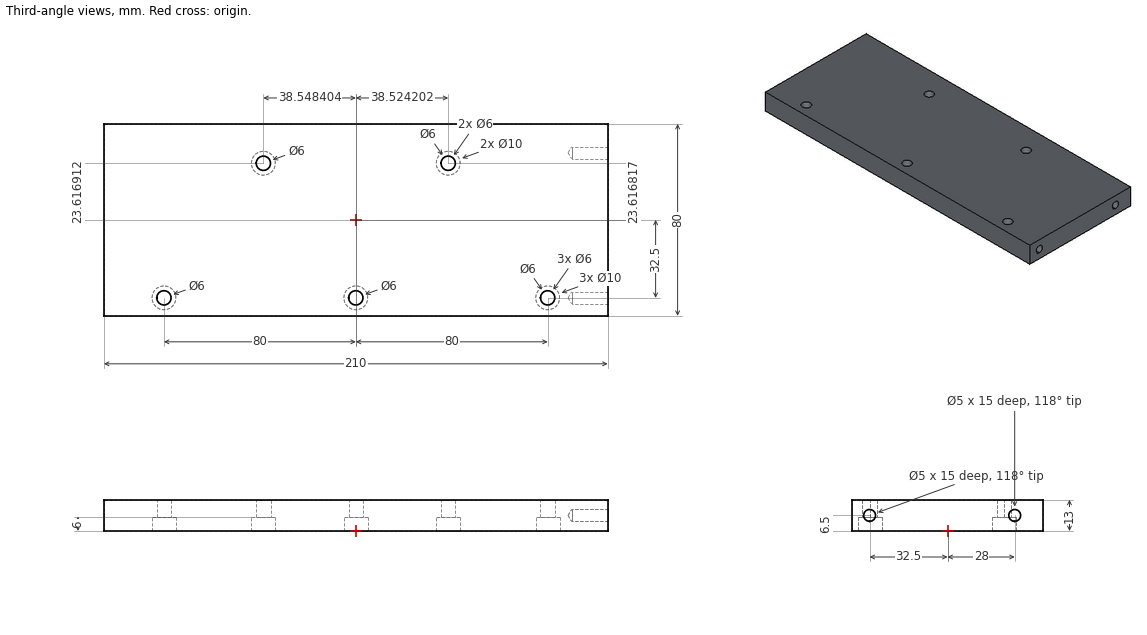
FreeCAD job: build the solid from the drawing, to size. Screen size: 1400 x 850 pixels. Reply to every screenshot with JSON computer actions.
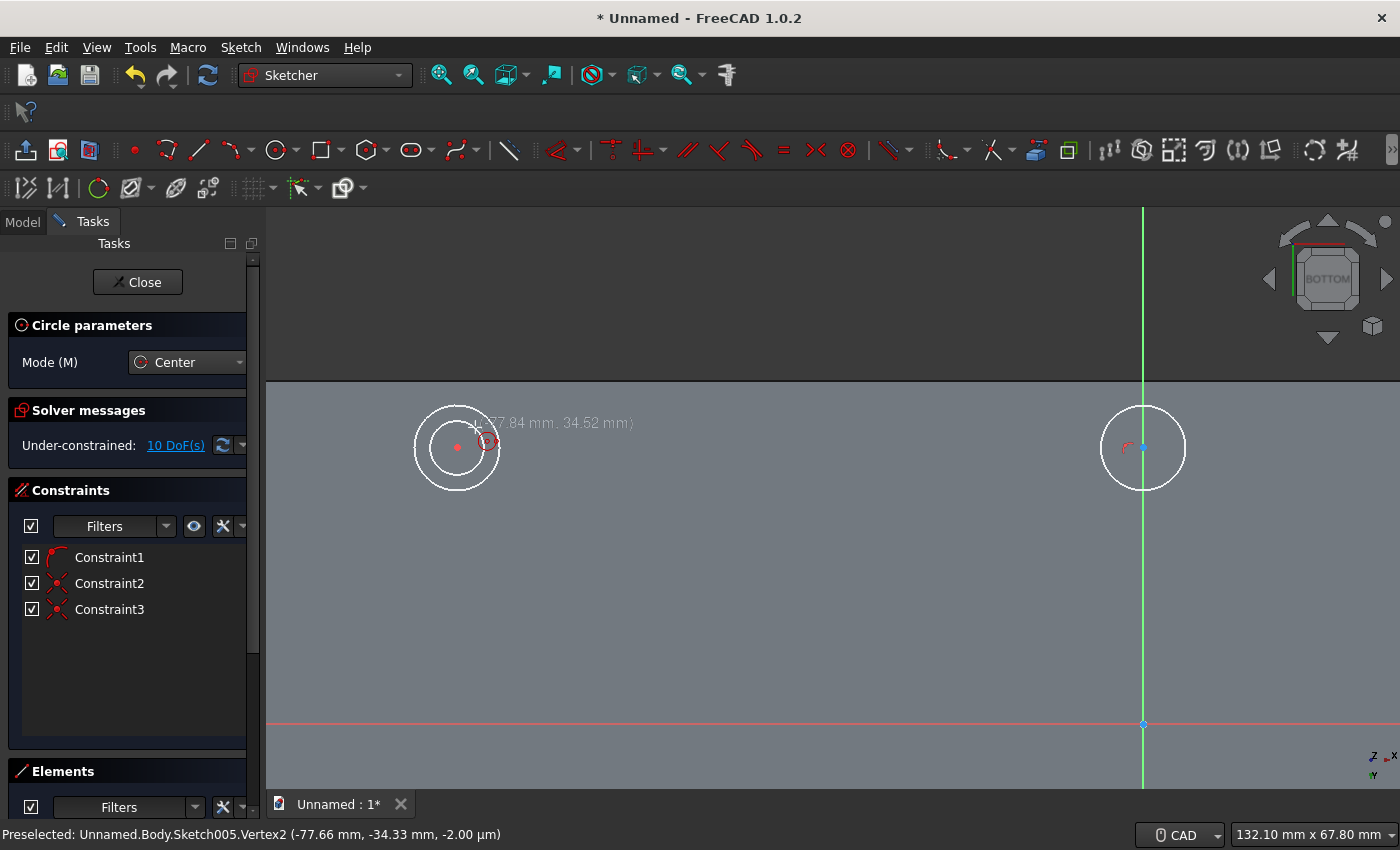
{"action": "left_click", "coordinate": [1143, 448]}
{"action": "left_click", "coordinate": [1161, 427]}
{"action": "key", "text": "Escape"}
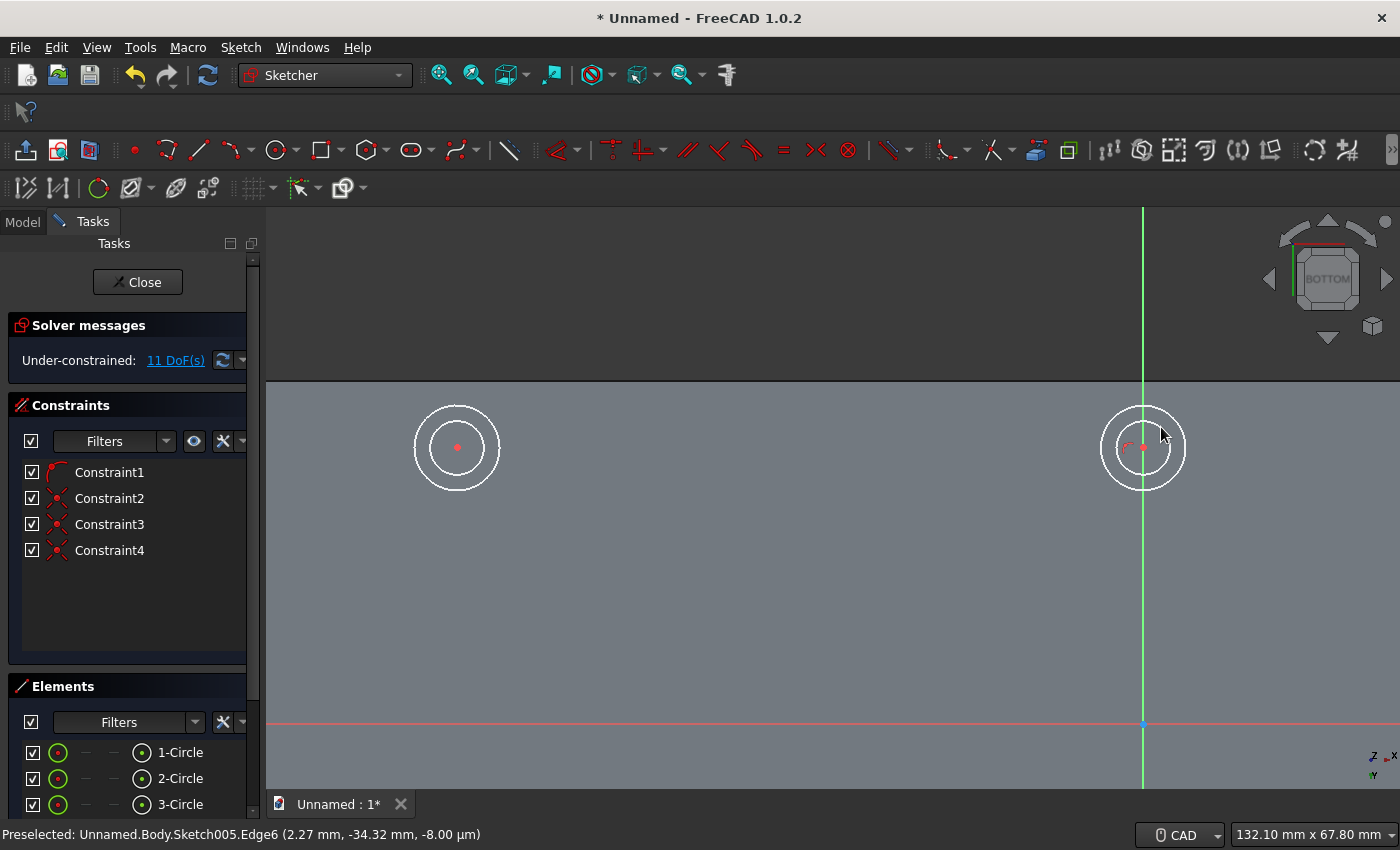
{"action": "scroll", "coordinate": [455, 445], "scroll_direction": "down", "scroll_amount": 4}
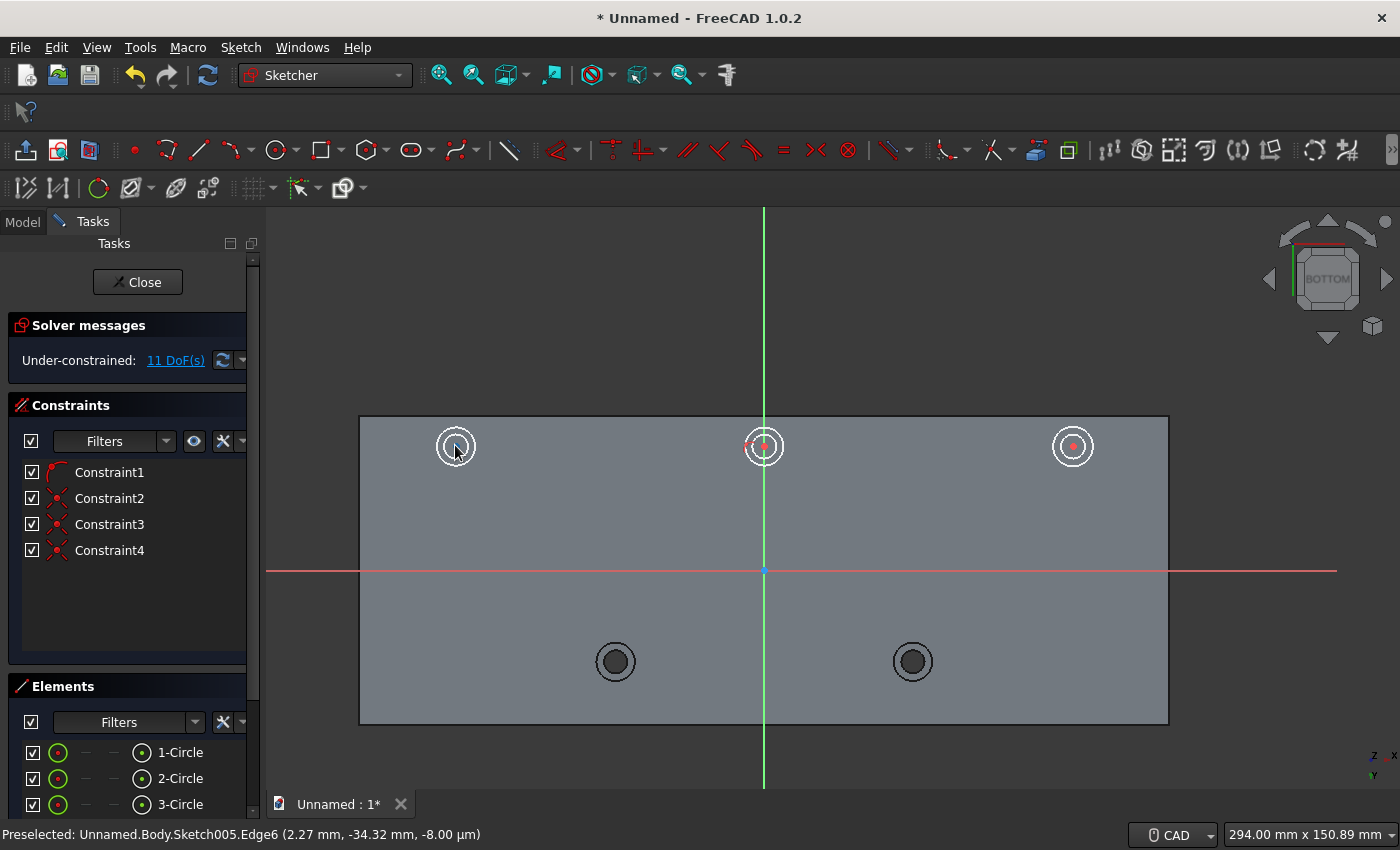
{"action": "scroll", "coordinate": [1087, 433], "scroll_direction": "up", "scroll_amount": 3}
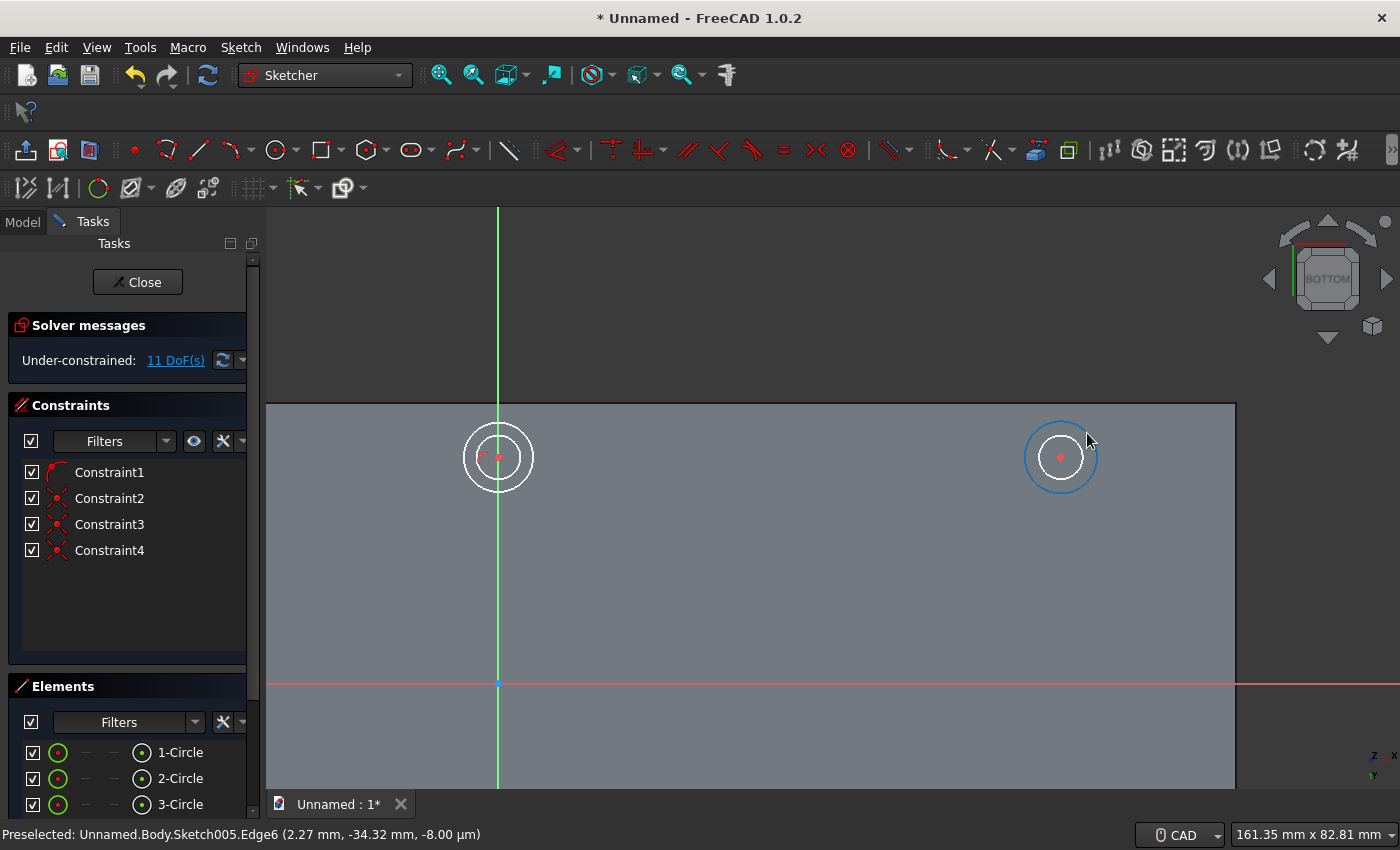
{"action": "left_click", "coordinate": [1086, 432]}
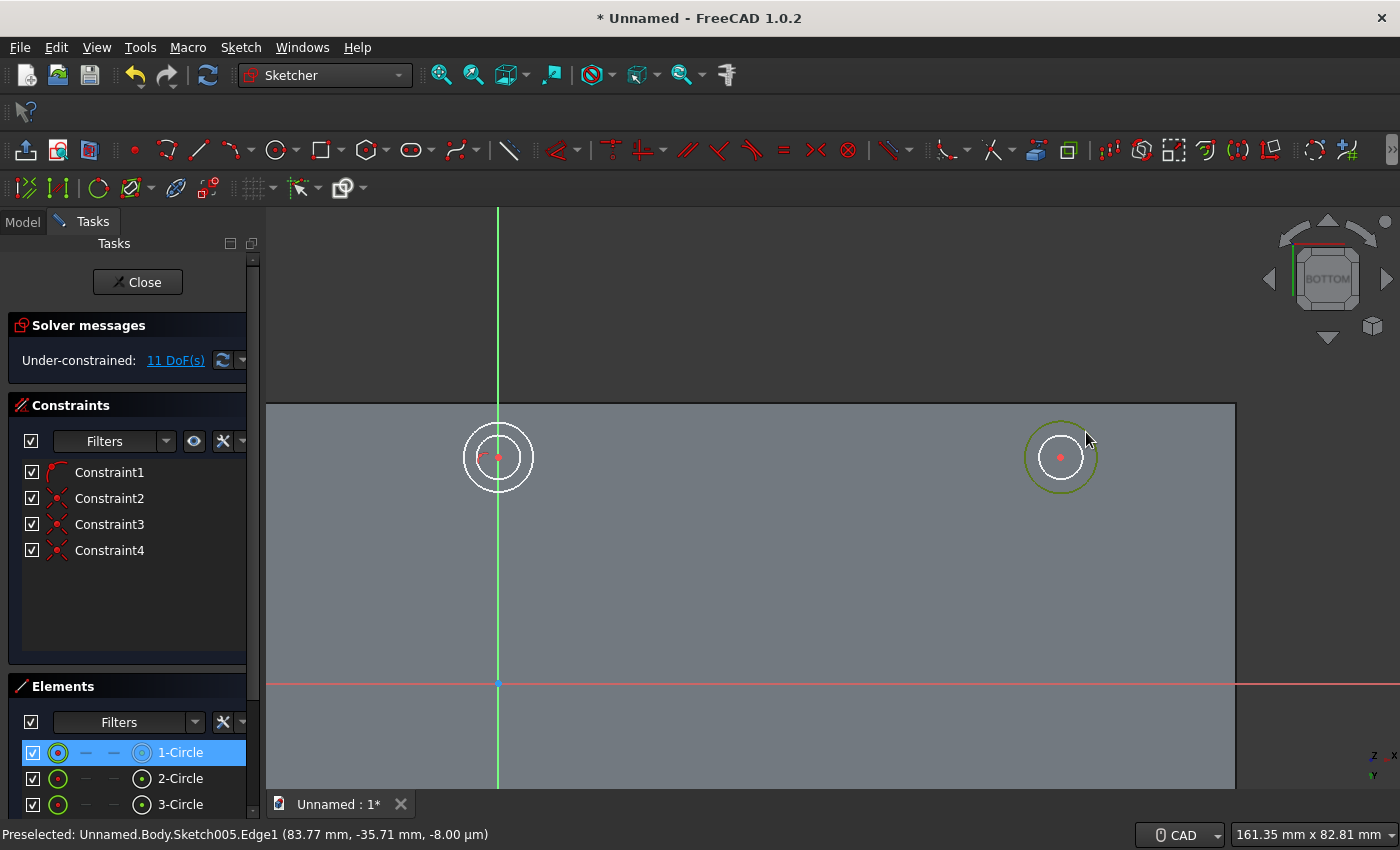
{"action": "scroll", "coordinate": [1088, 432], "scroll_direction": "down", "scroll_amount": 3}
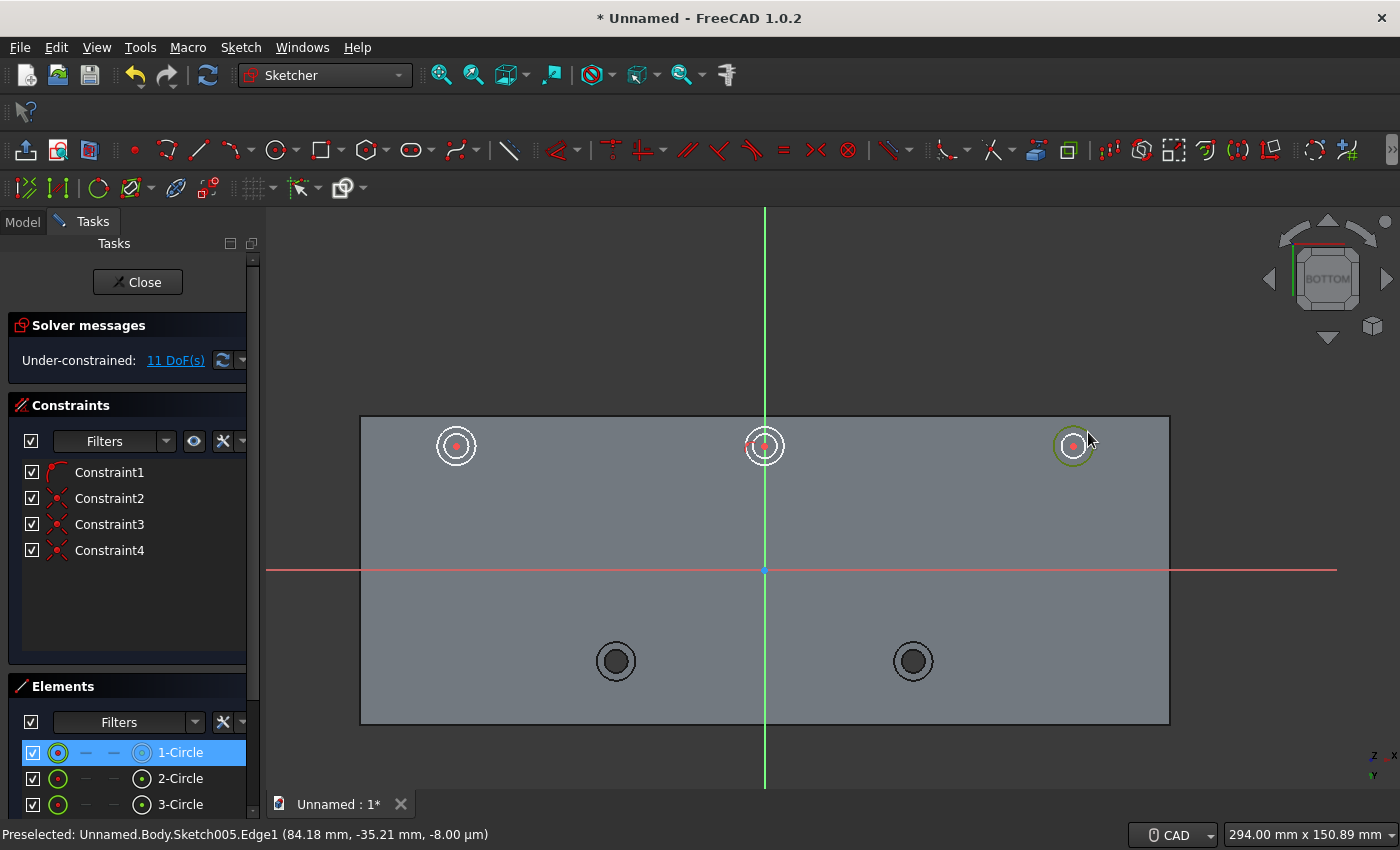
{"action": "scroll", "coordinate": [470, 433], "scroll_direction": "up", "scroll_amount": 4}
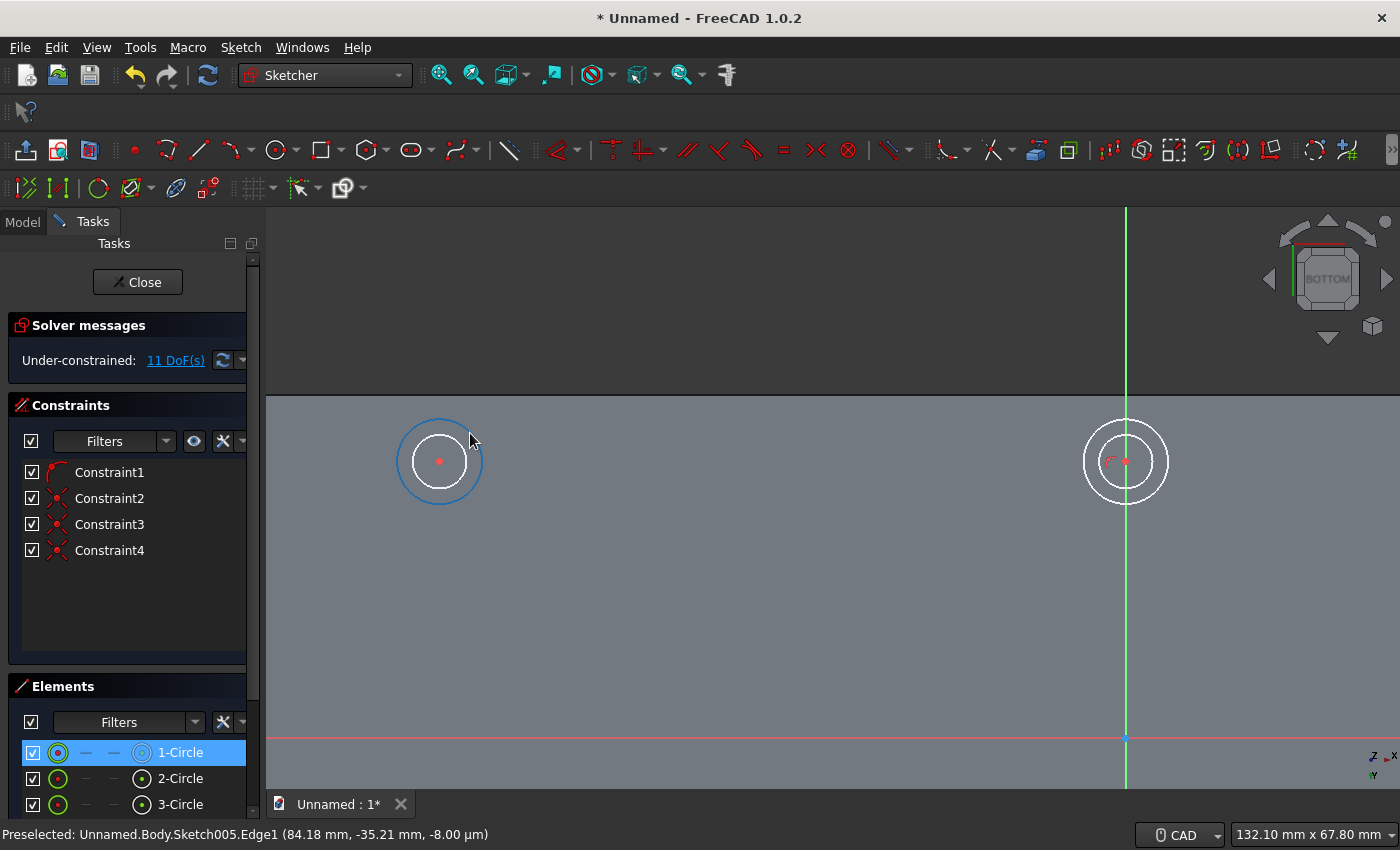
{"action": "left_click", "coordinate": [470, 432]}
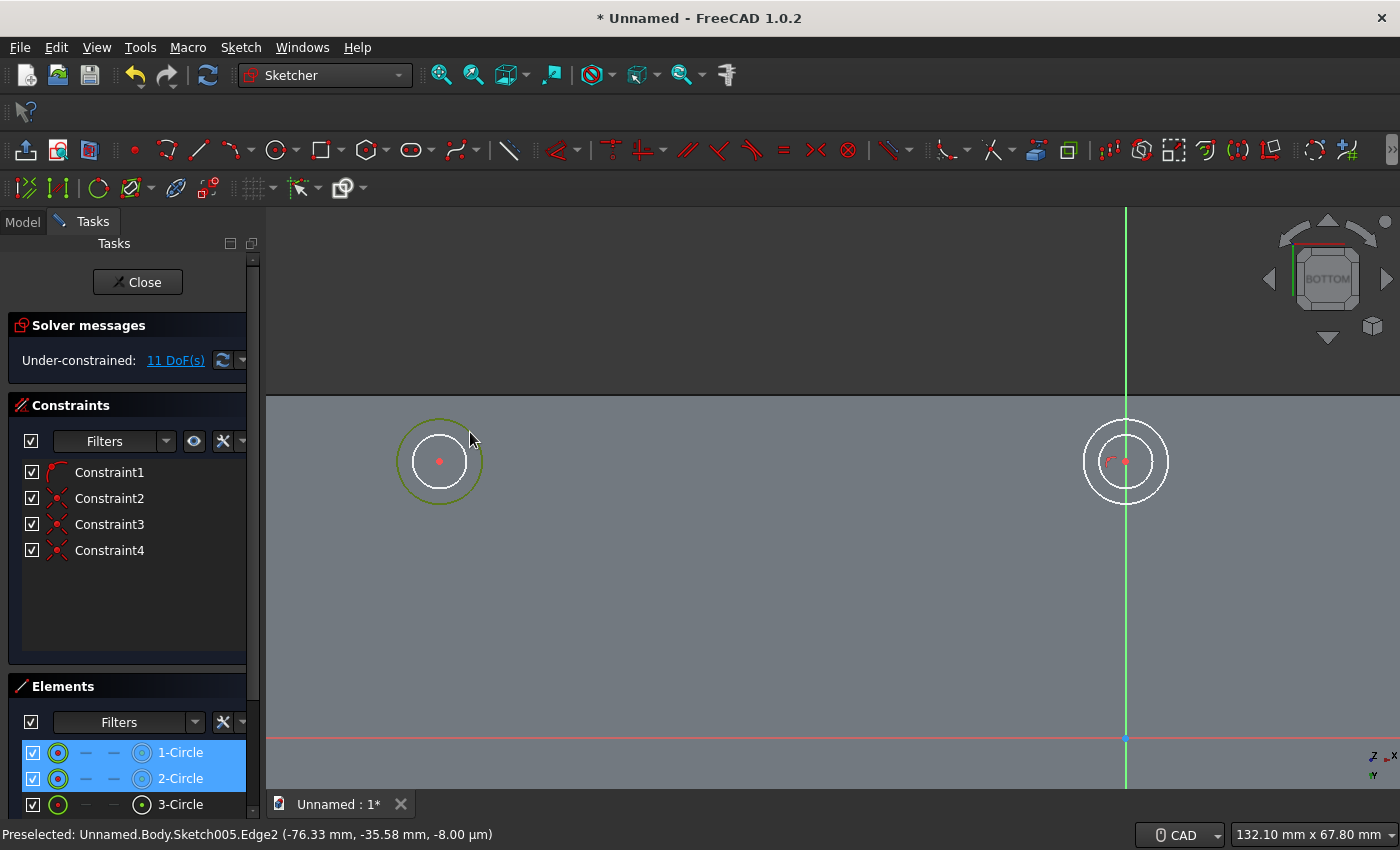
{"action": "left_click", "coordinate": [1156, 432]}